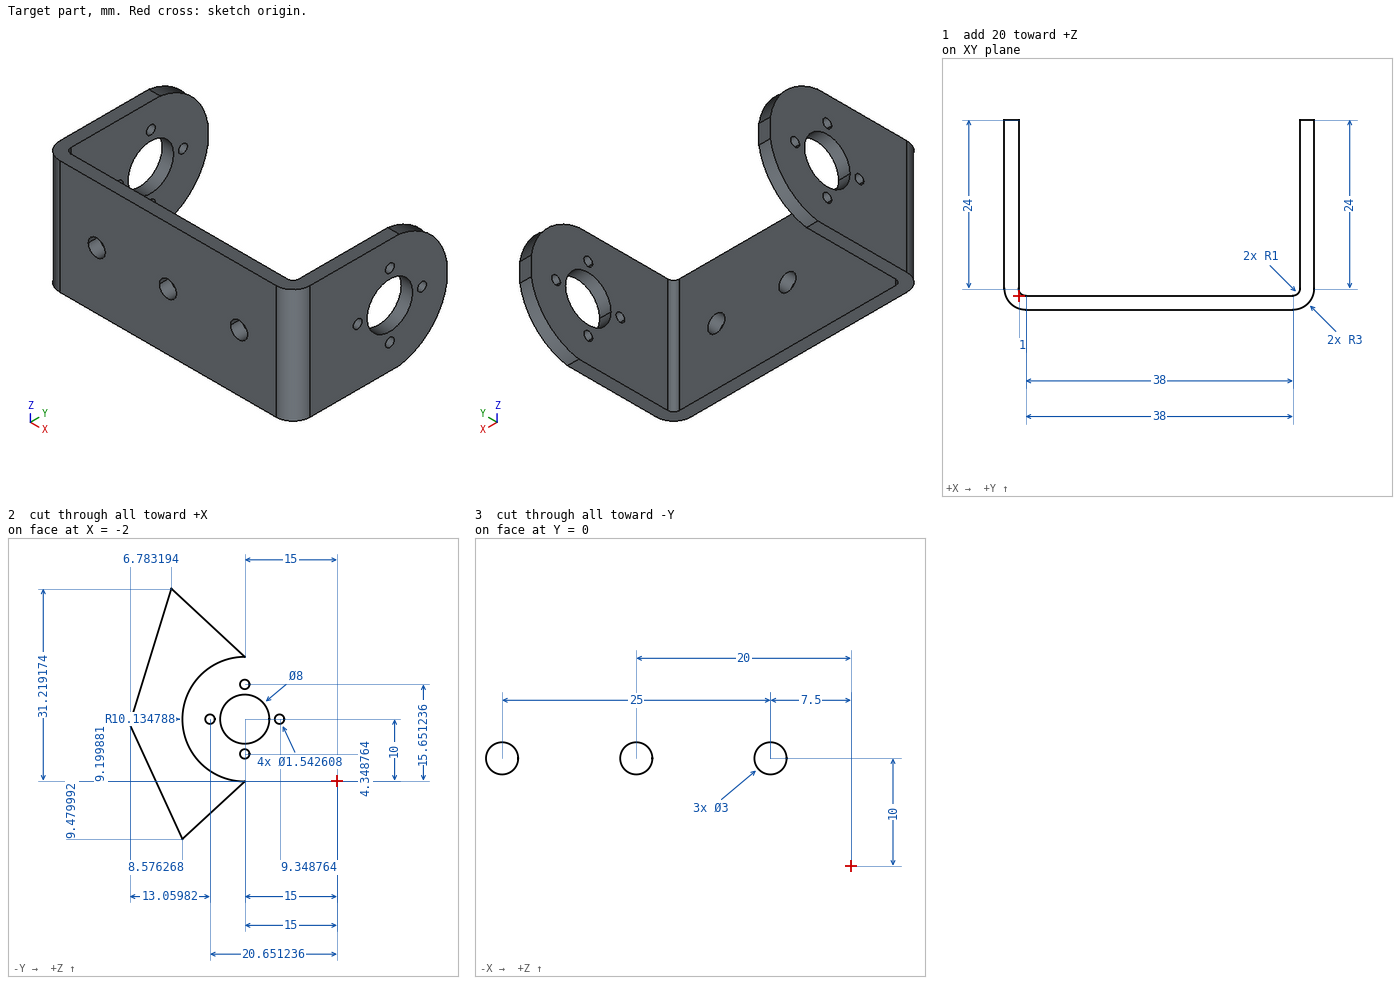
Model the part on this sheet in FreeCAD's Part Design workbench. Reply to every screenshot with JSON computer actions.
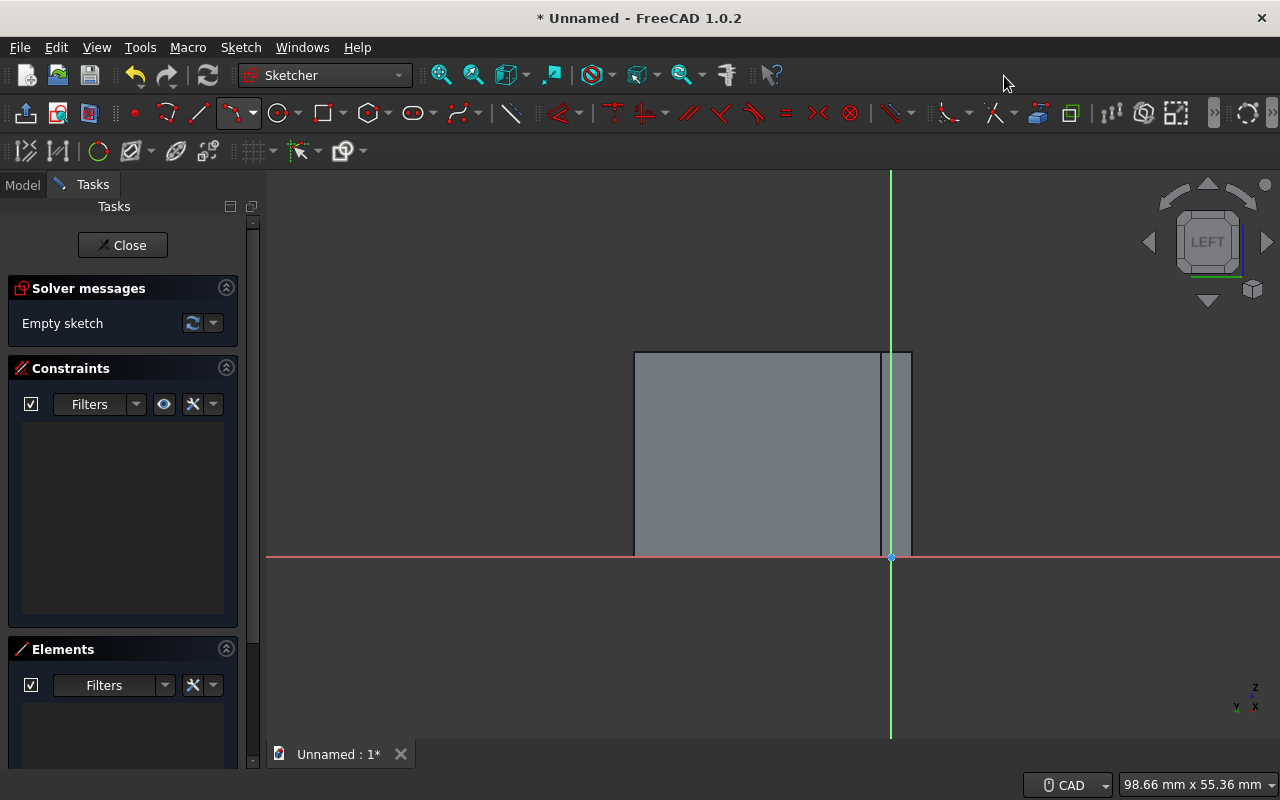
{"action": "left_click", "coordinate": [737, 350]}
{"action": "left_click", "coordinate": [614, 236]}
{"action": "left_click", "coordinate": [545, 463]}
{"action": "left_click", "coordinate": [633, 655]}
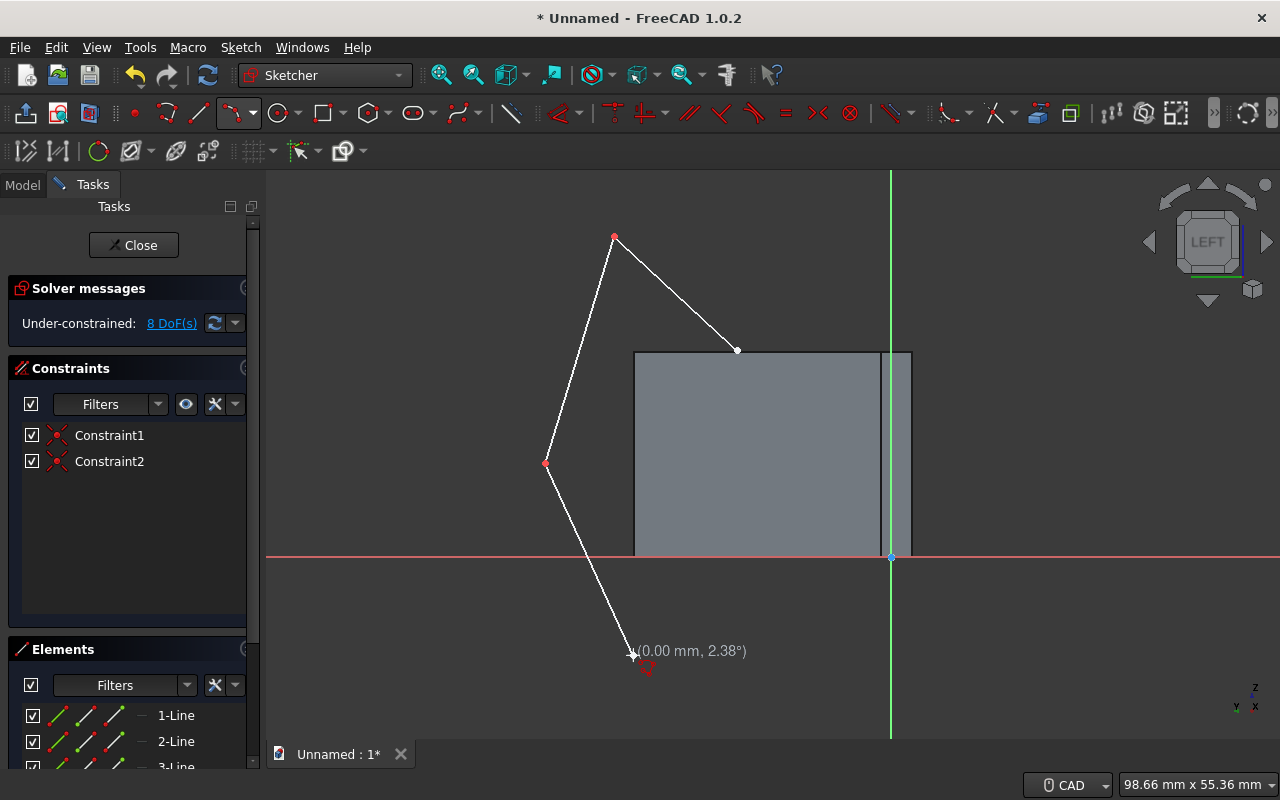
{"action": "scroll", "coordinate": [737, 559], "scroll_direction": "up", "scroll_amount": 13}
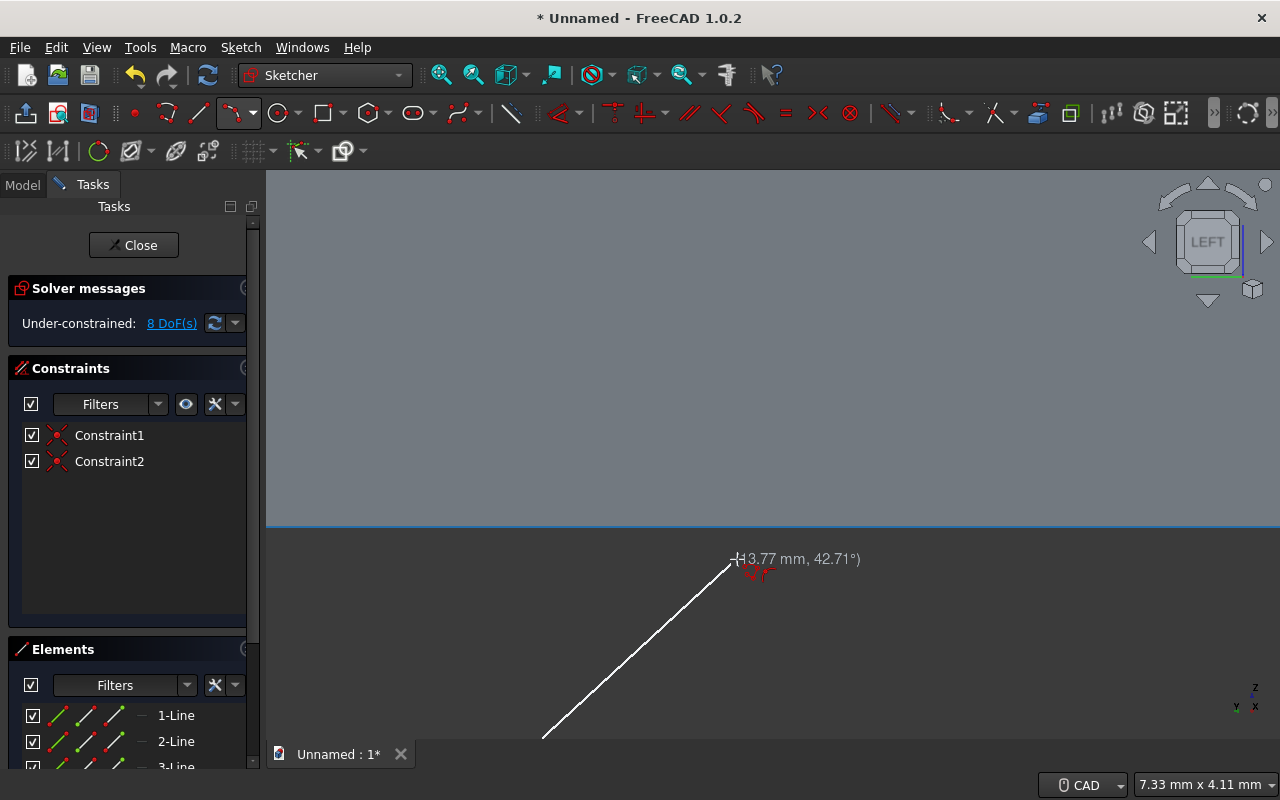
{"action": "left_click", "coordinate": [732, 546]}
{"action": "right_click", "coordinate": [732, 546]}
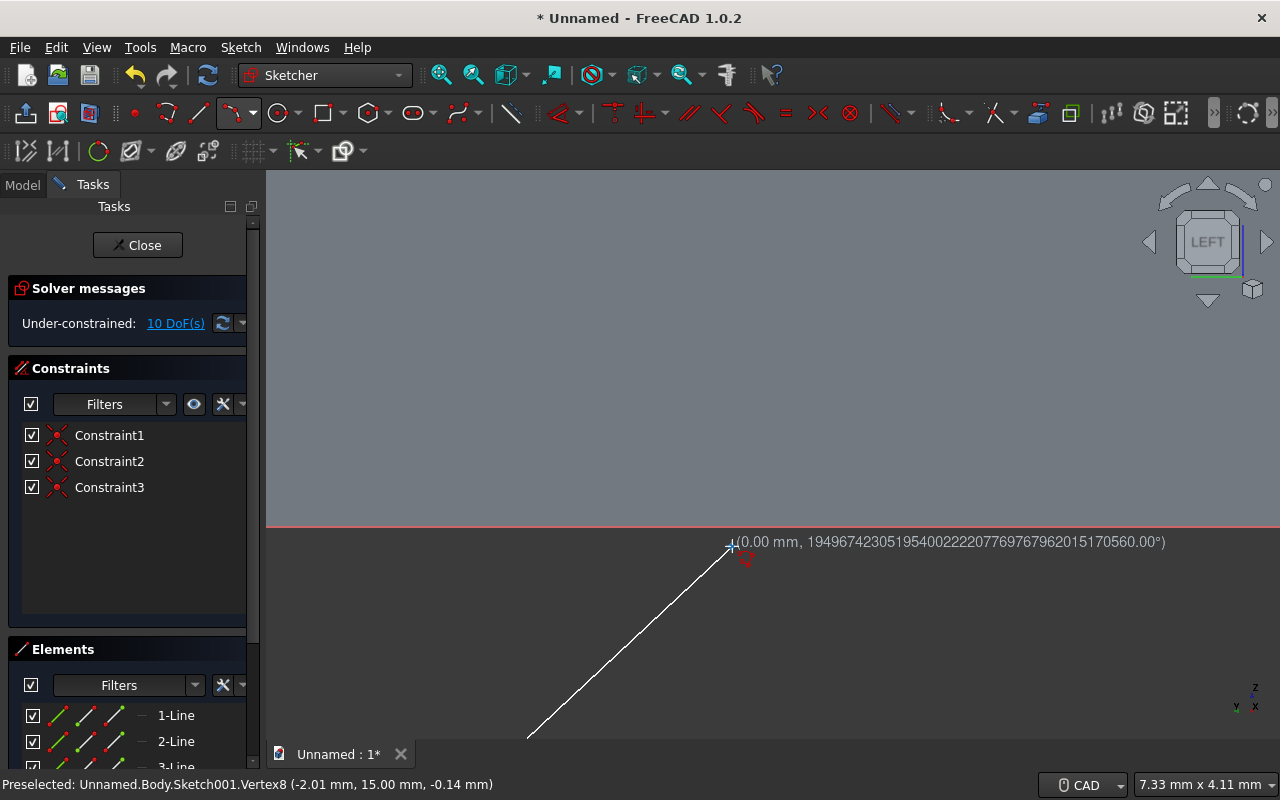
{"action": "left_click", "coordinate": [232, 114]}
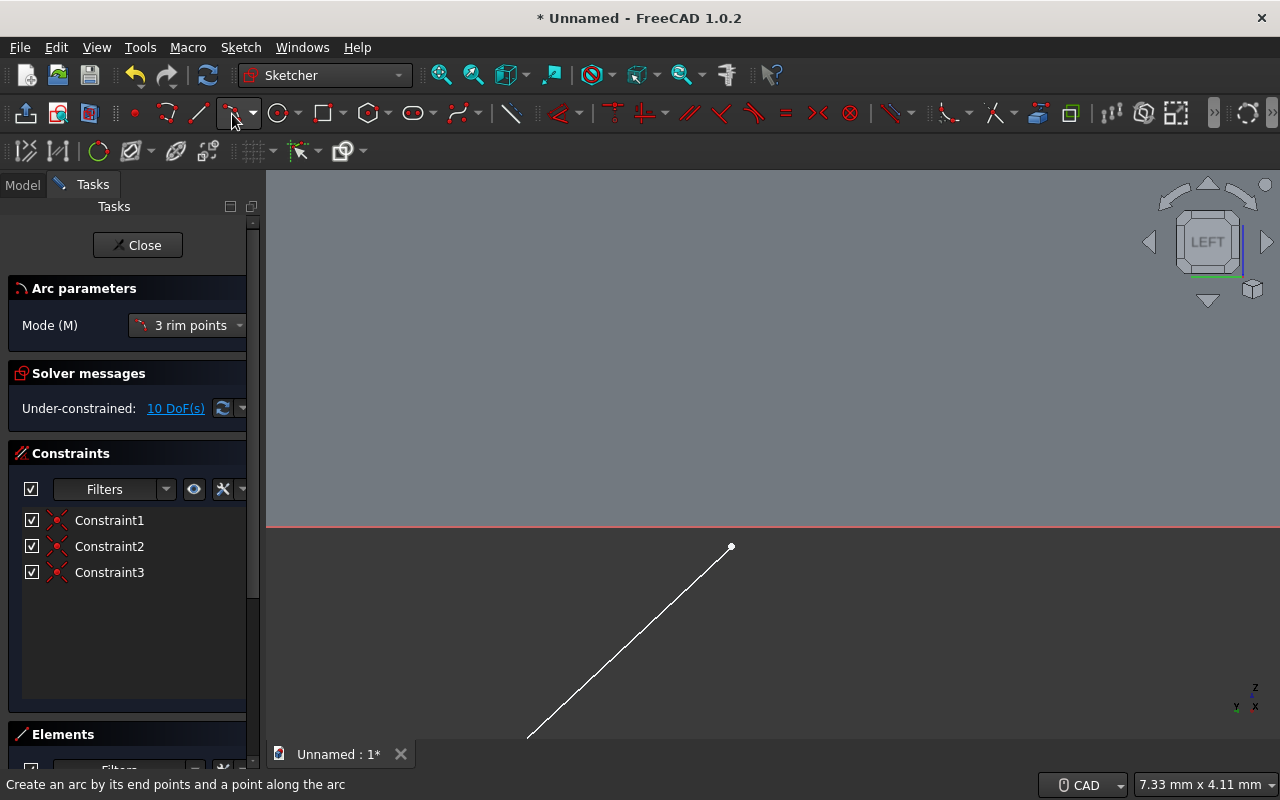
{"action": "left_click", "coordinate": [732, 547]}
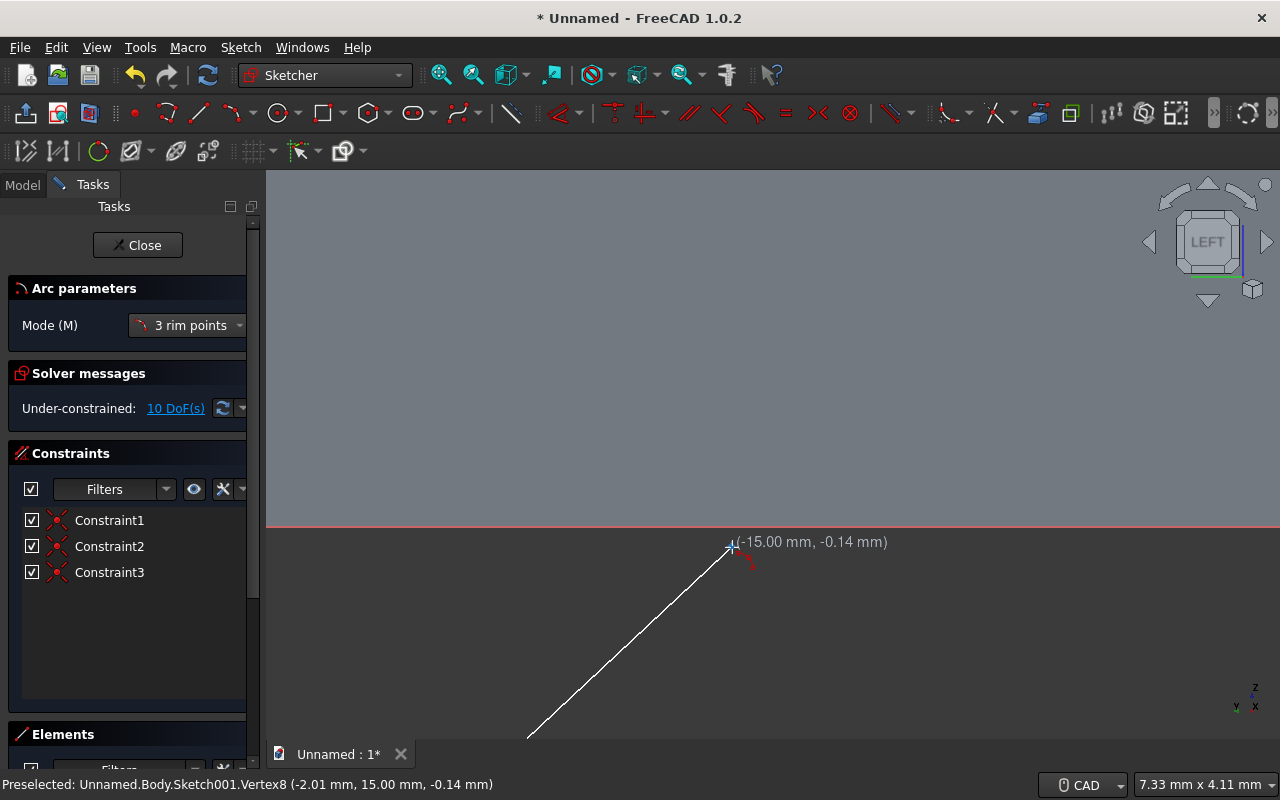
{"action": "scroll", "coordinate": [719, 547], "scroll_direction": "down", "scroll_amount": 14}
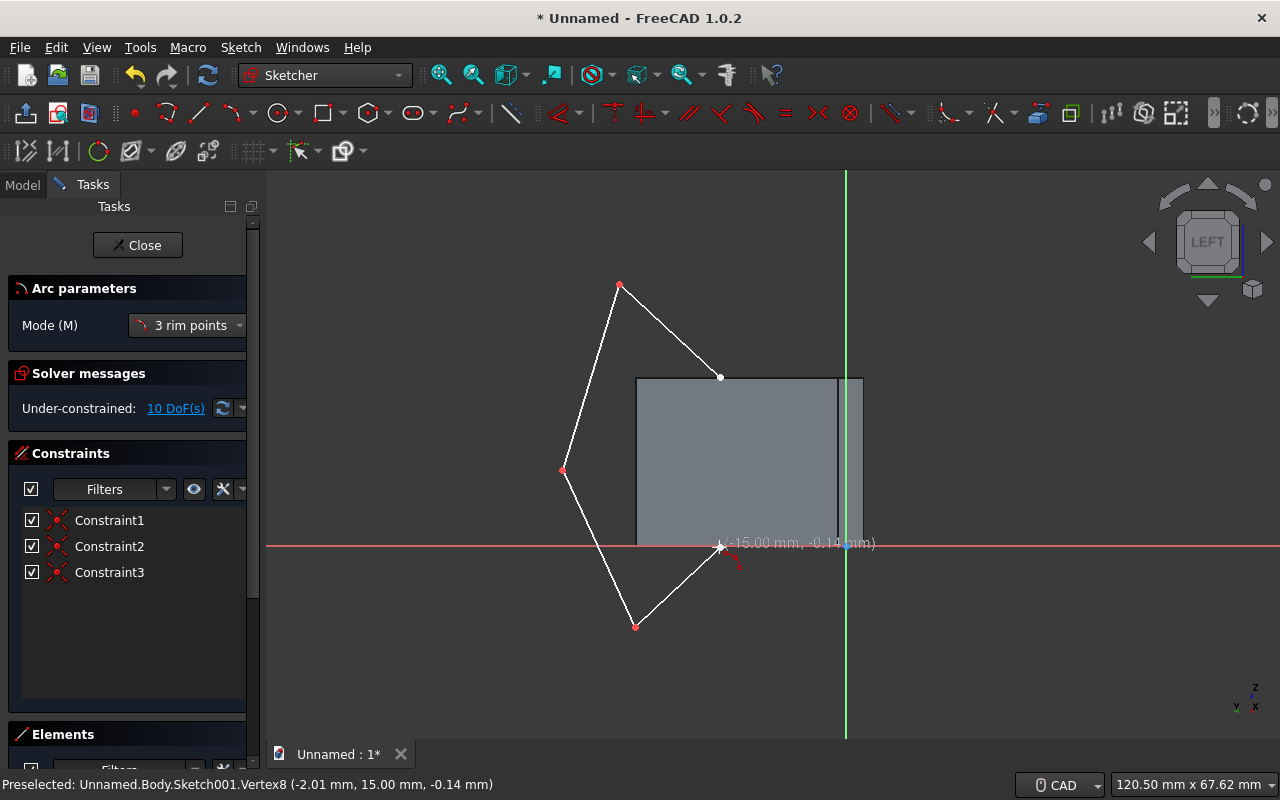
{"action": "left_click", "coordinate": [720, 378]}
{"action": "left_click", "coordinate": [635, 462]}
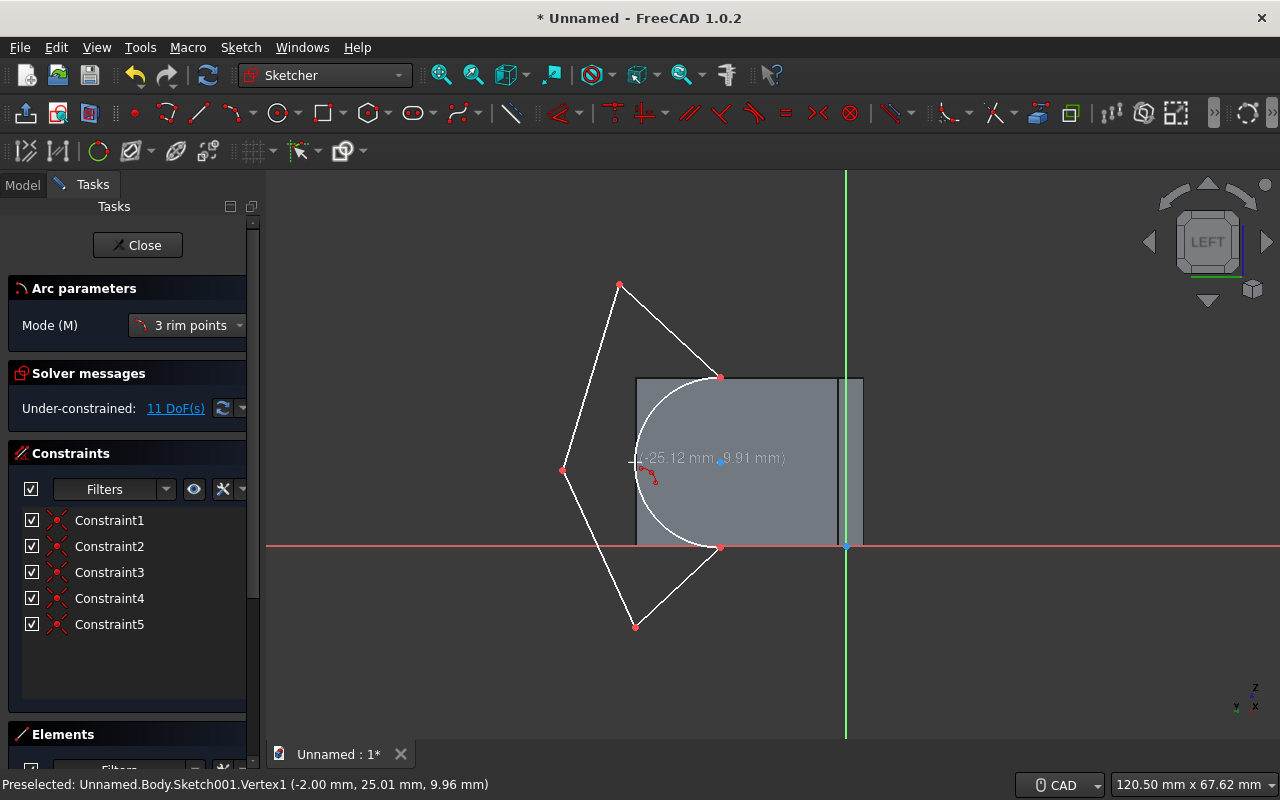
{"action": "left_click", "coordinate": [278, 114]}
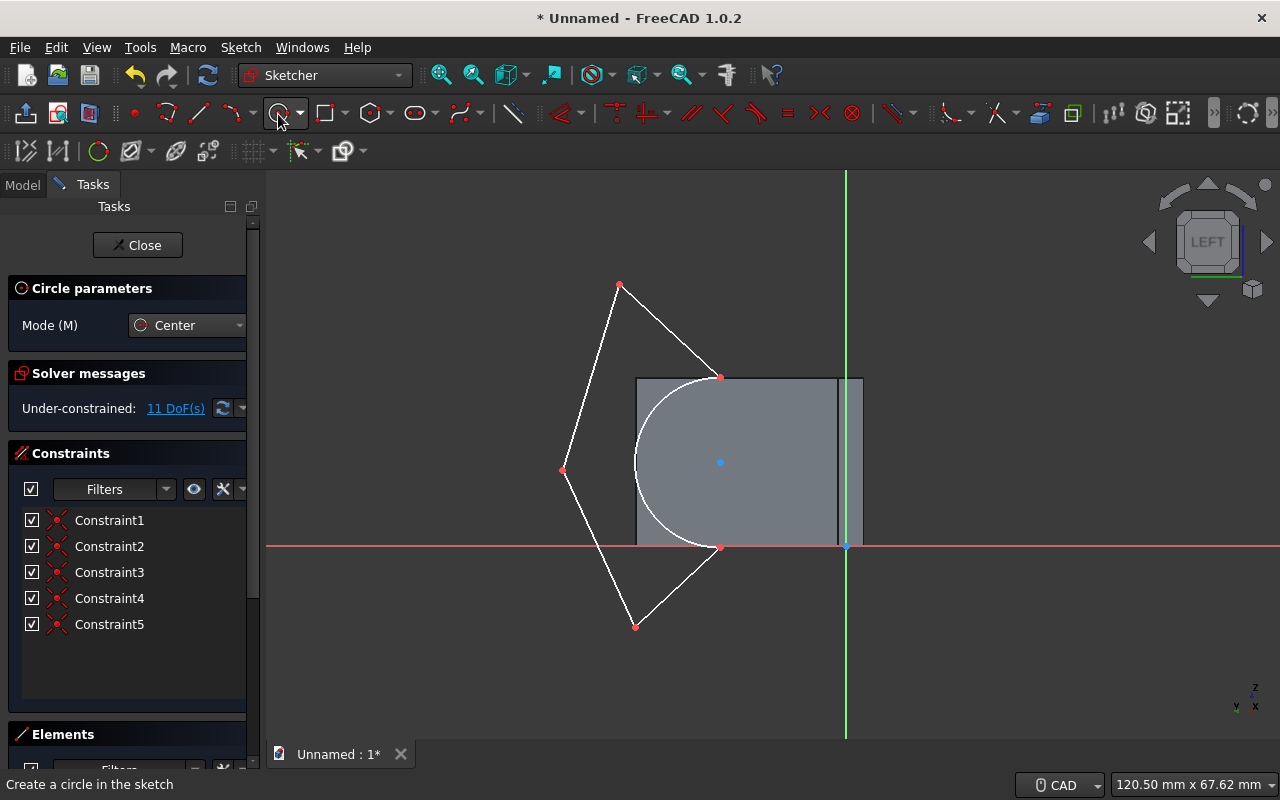
{"action": "left_click", "coordinate": [720, 462]}
{"action": "mouse_move", "coordinate": [744, 438]}